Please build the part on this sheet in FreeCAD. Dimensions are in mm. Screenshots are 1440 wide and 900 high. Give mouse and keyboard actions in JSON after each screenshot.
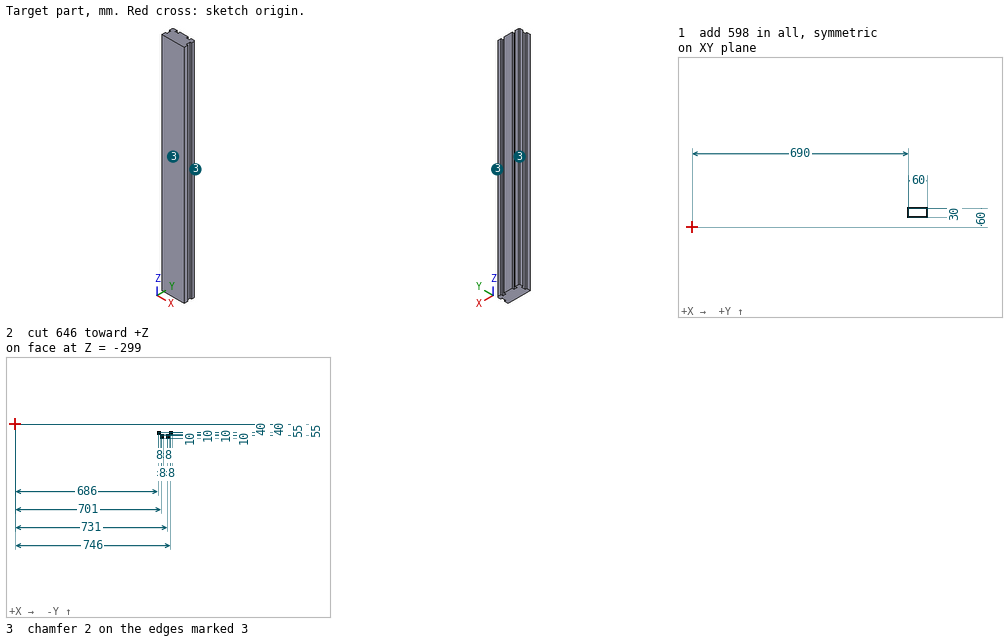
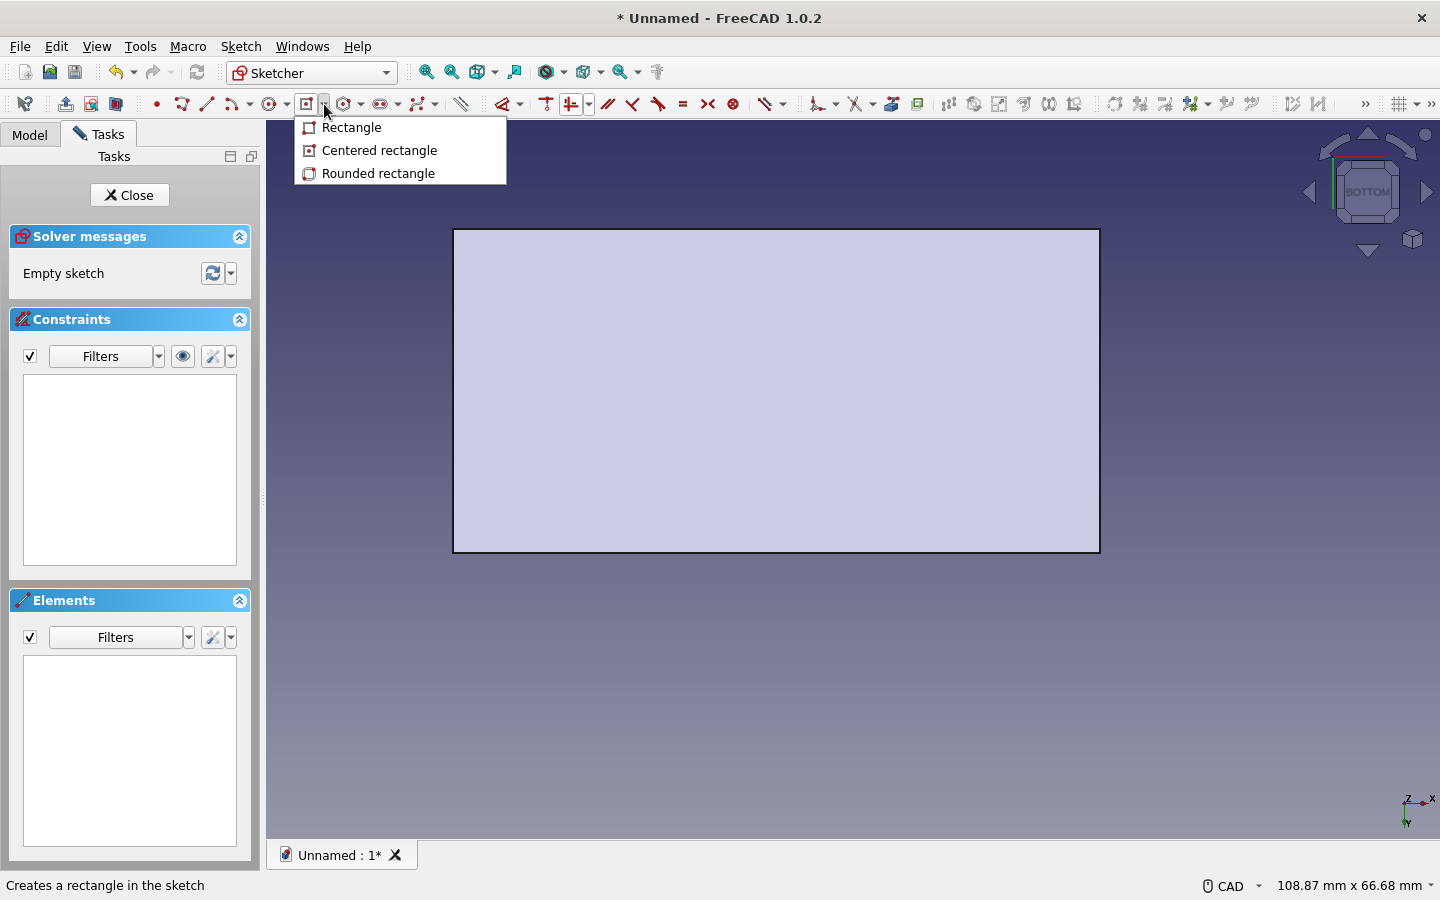
{"action": "left_click", "coordinate": [400, 128]}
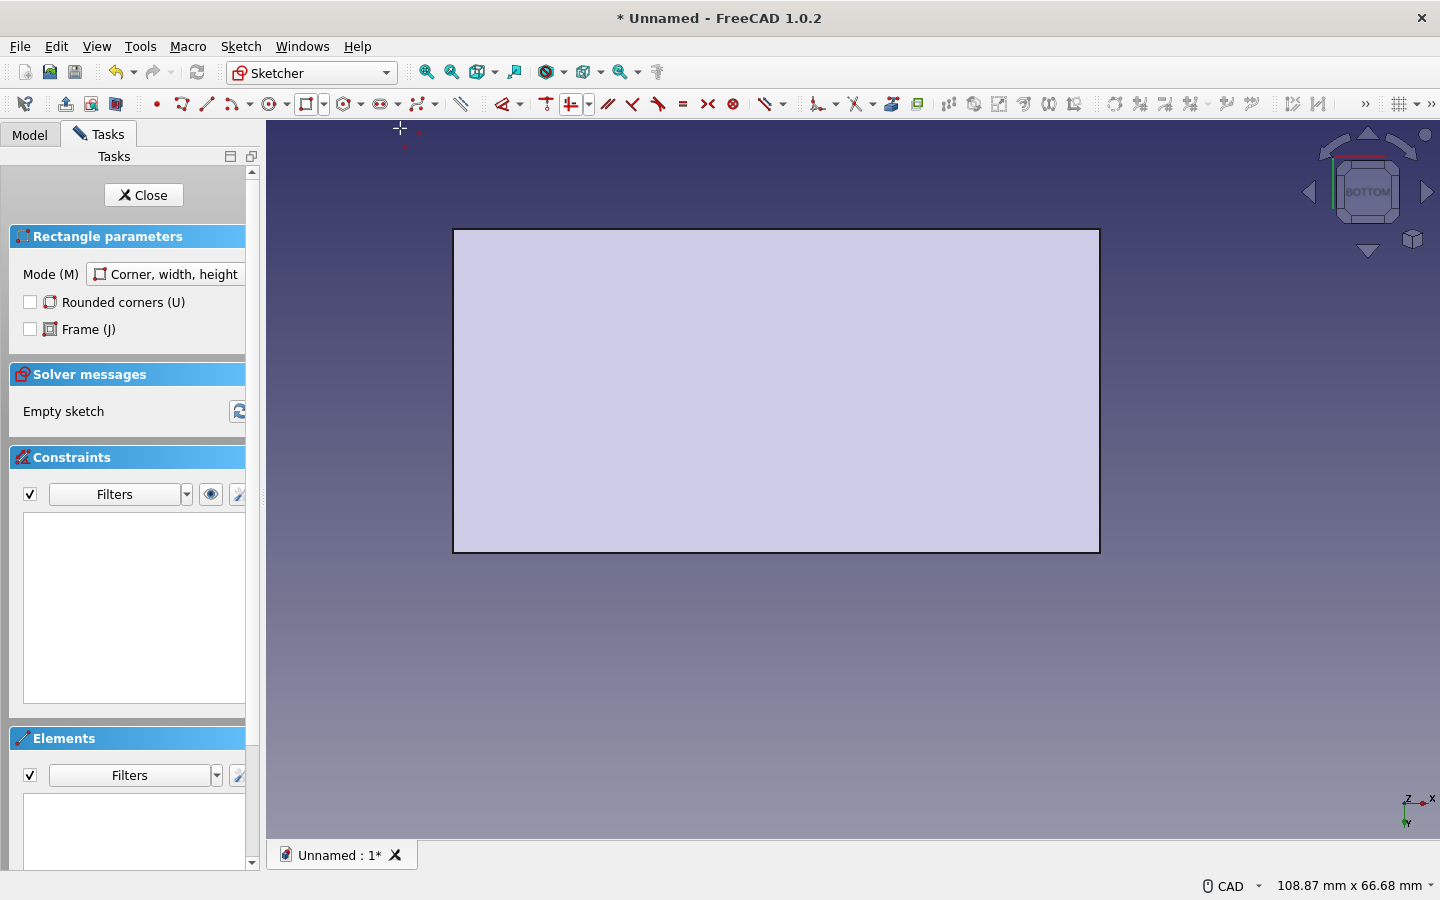
{"action": "left_click", "coordinate": [895, 499]}
{"action": "left_click", "coordinate": [982, 607]}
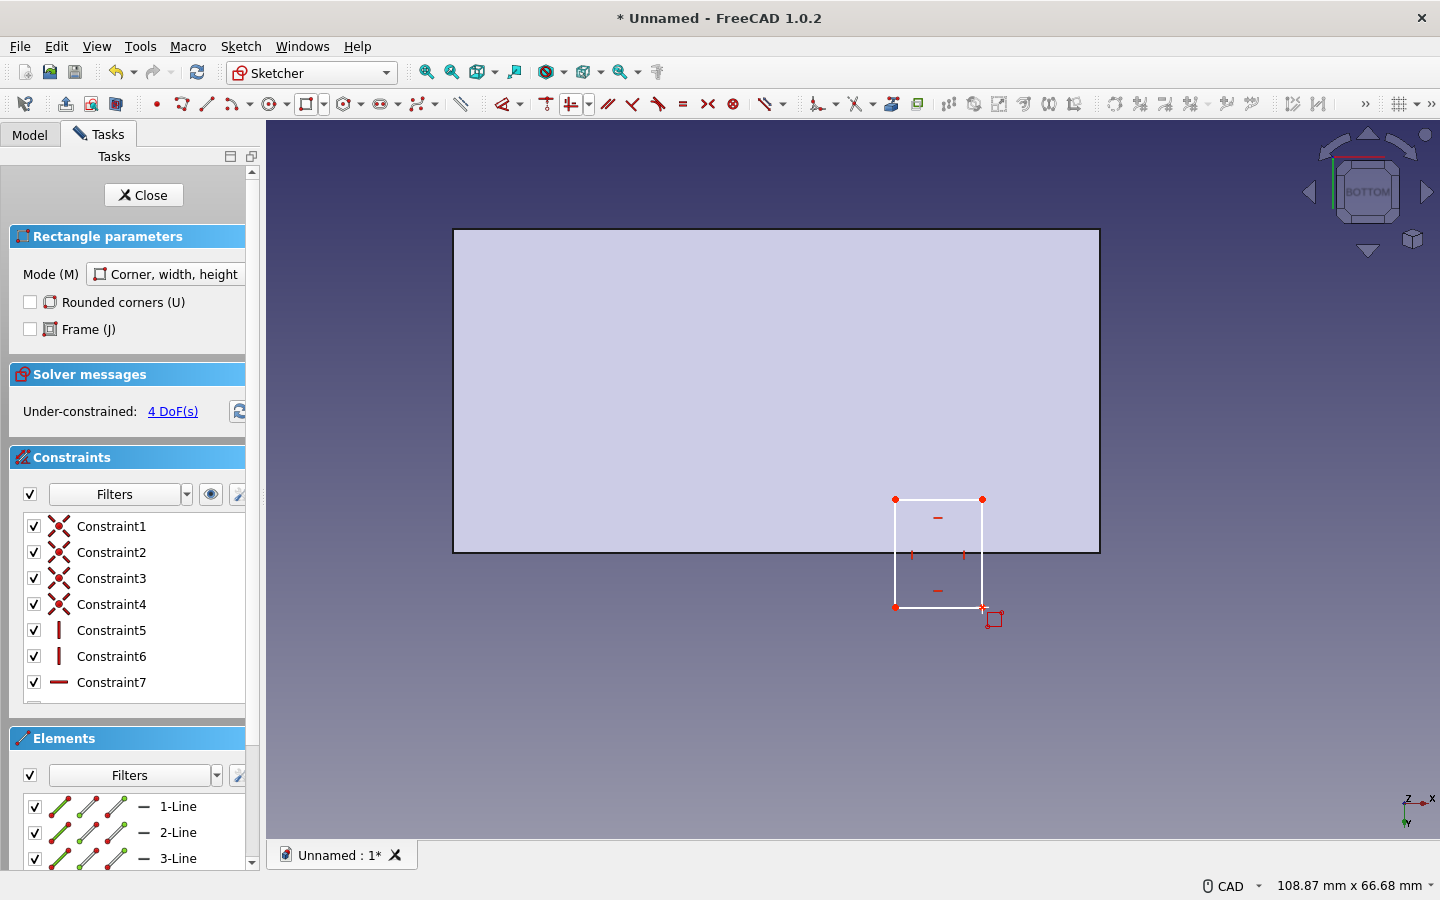
{"action": "left_click", "coordinate": [1057, 337]}
{"action": "left_click", "coordinate": [1143, 445]}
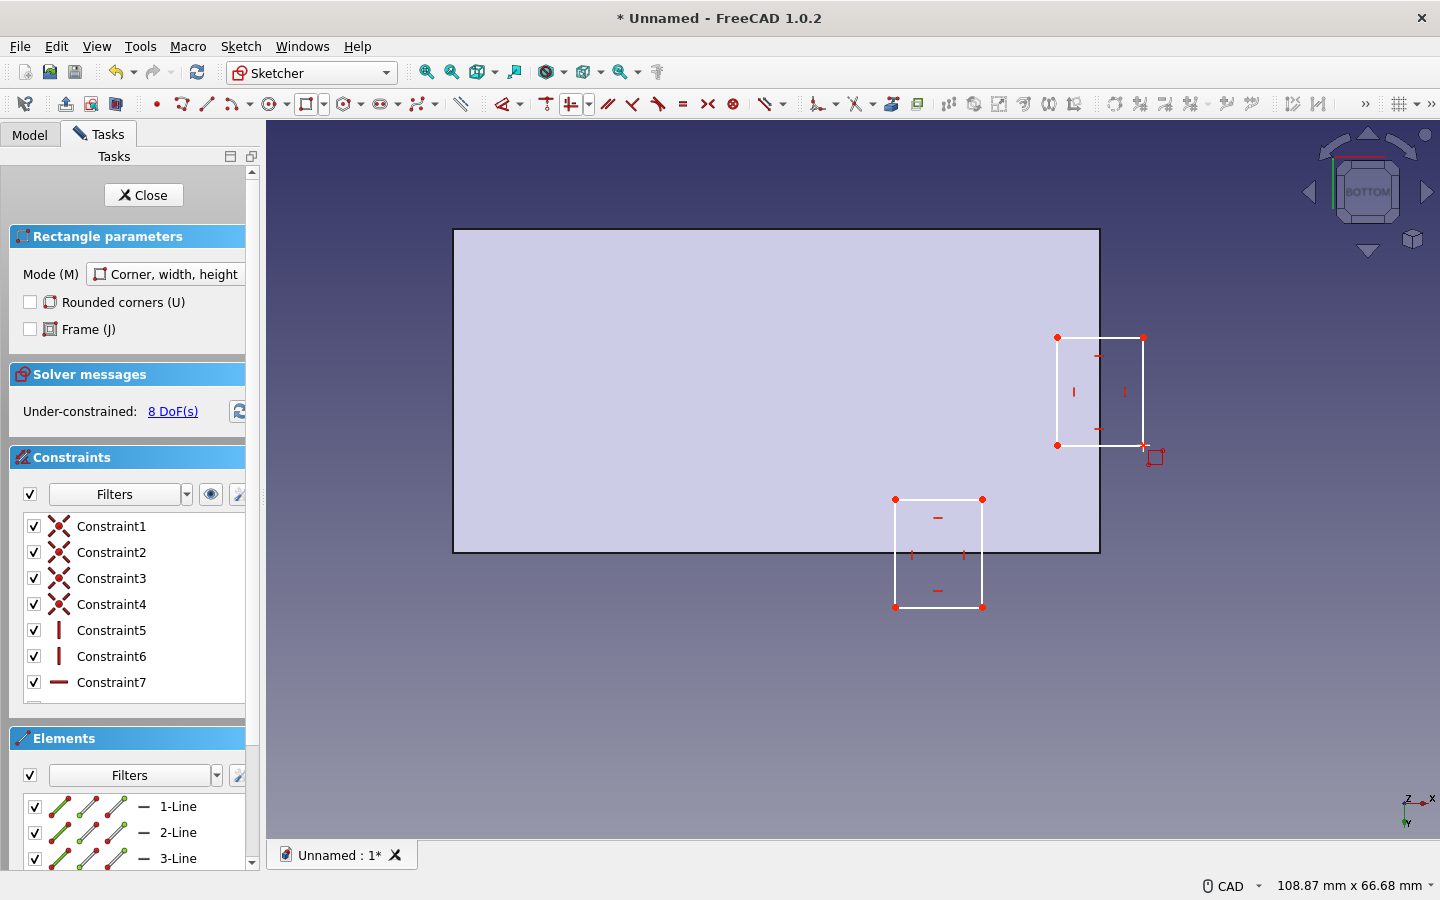
{"action": "left_click", "coordinate": [410, 337]}
{"action": "left_click", "coordinate": [496, 445]}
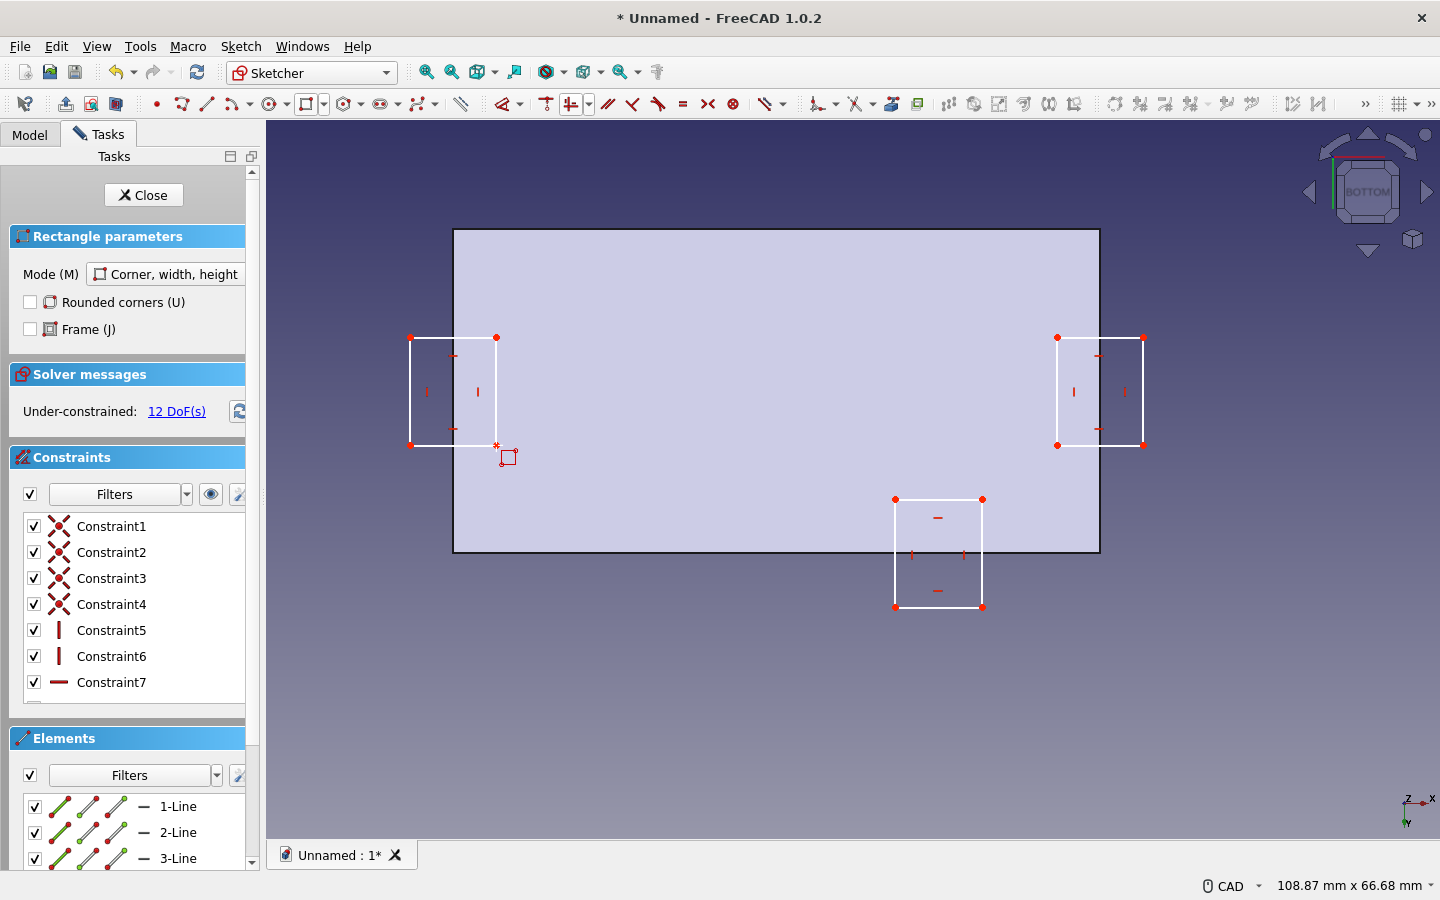
{"action": "left_click", "coordinate": [572, 499]}
{"action": "left_click", "coordinate": [658, 607]}
{"action": "key", "text": "Escape"}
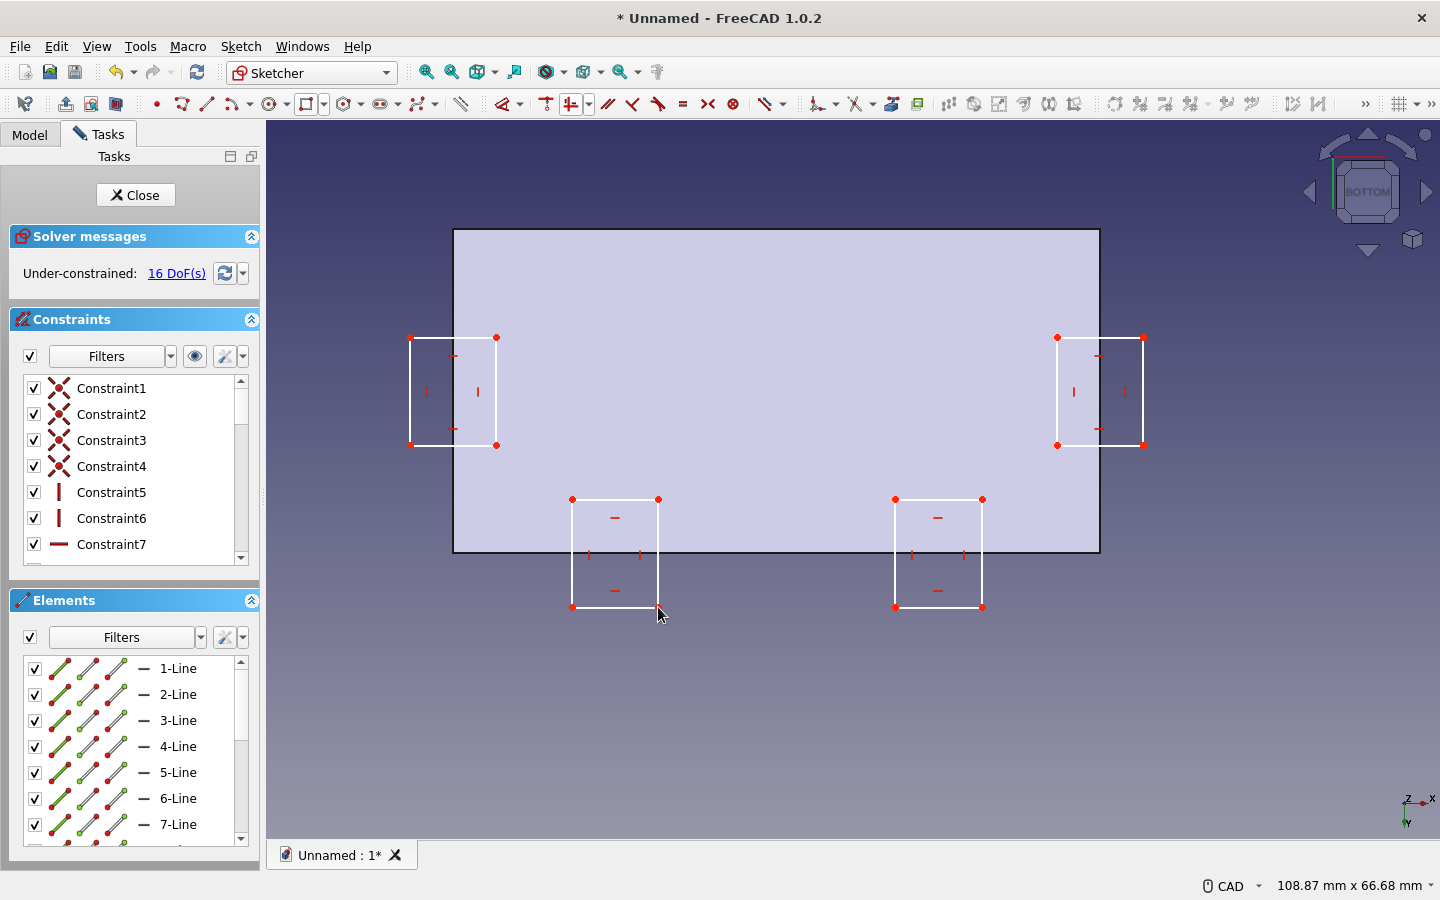
{"action": "left_click", "coordinate": [502, 104]}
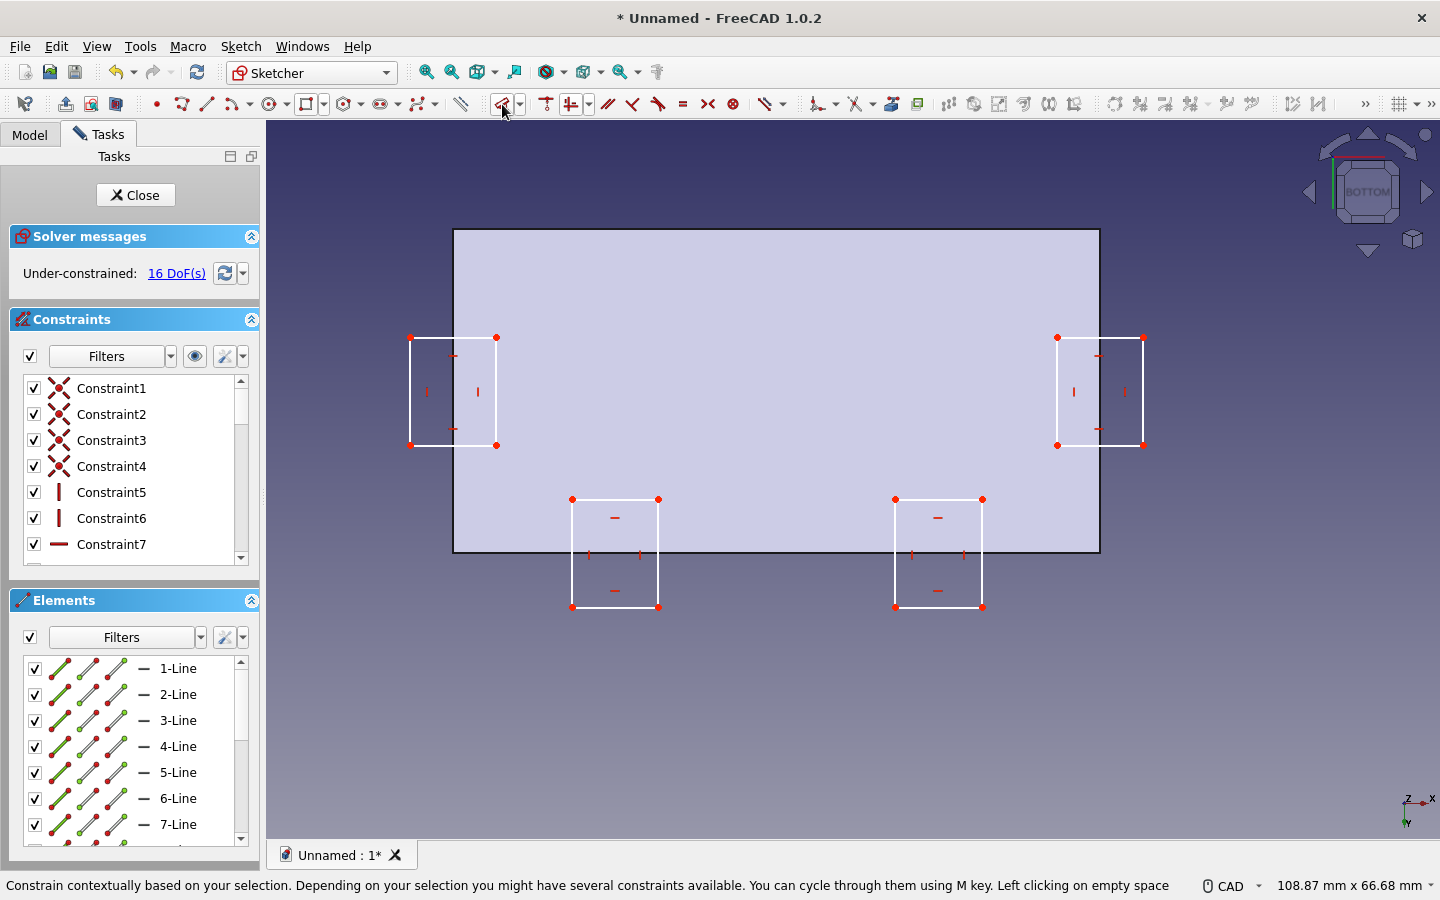
{"action": "left_click", "coordinate": [921, 608]}
{"action": "left_click", "coordinate": [938, 642]}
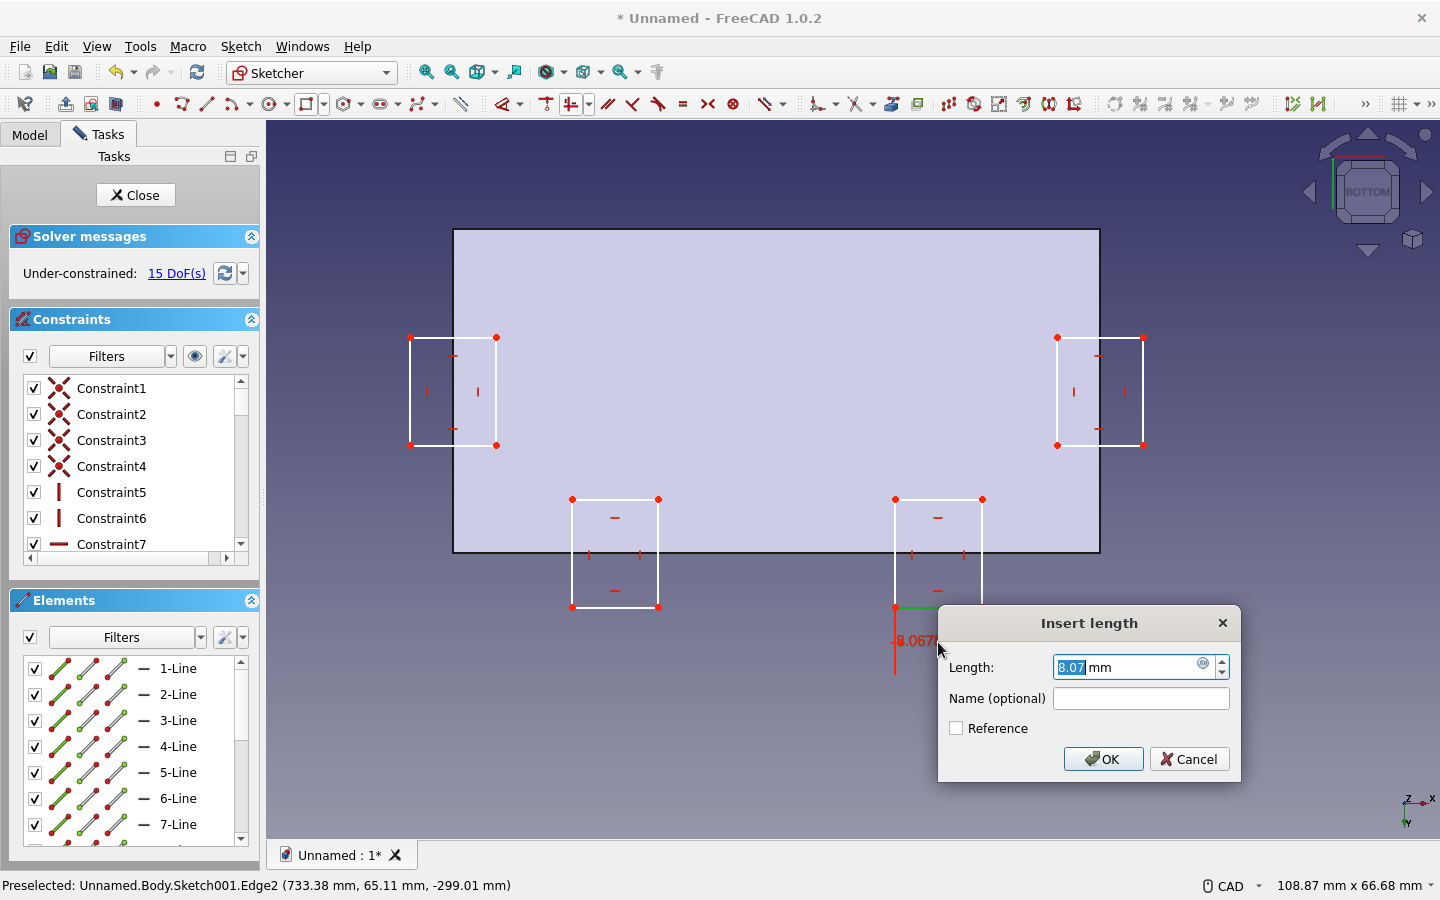
{"action": "type", "text": "8"}
{"action": "key", "text": "Return"}